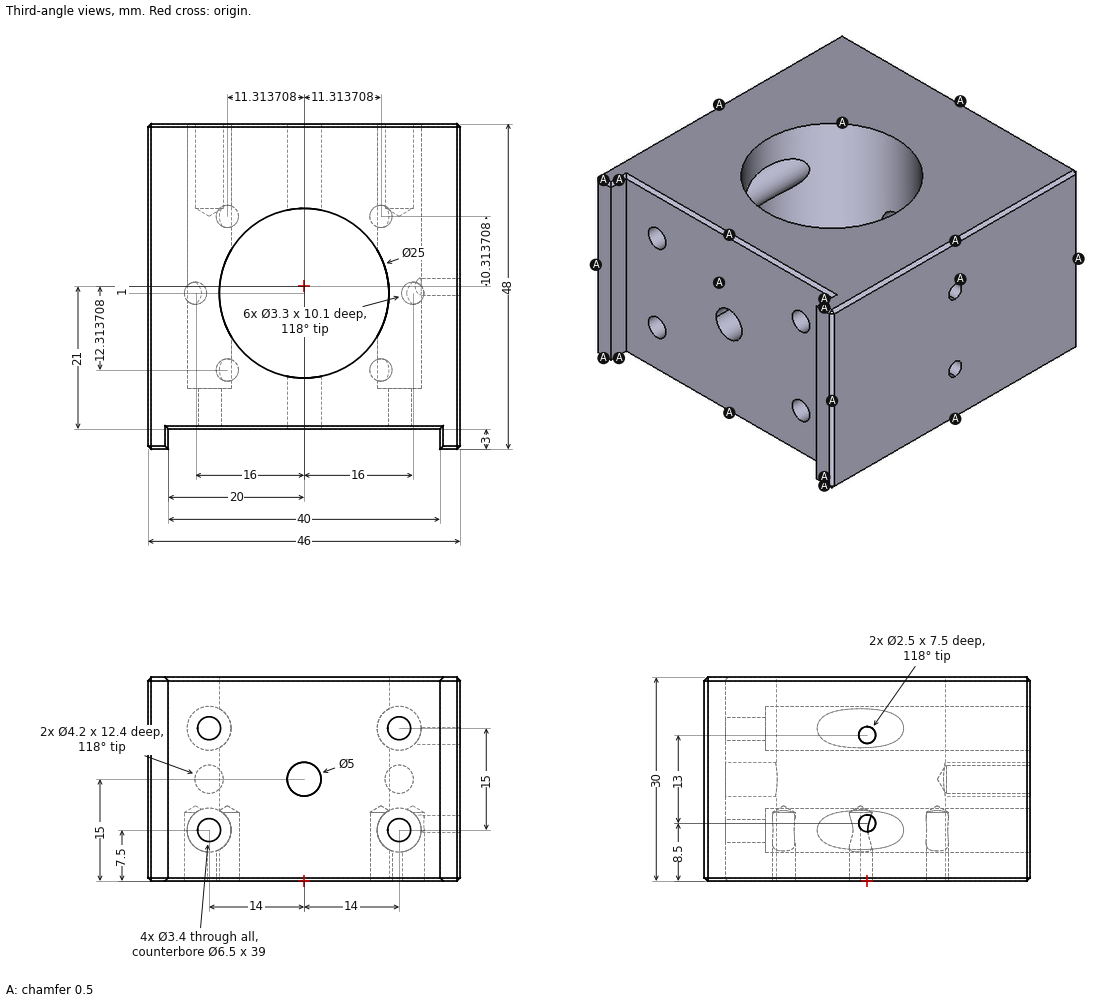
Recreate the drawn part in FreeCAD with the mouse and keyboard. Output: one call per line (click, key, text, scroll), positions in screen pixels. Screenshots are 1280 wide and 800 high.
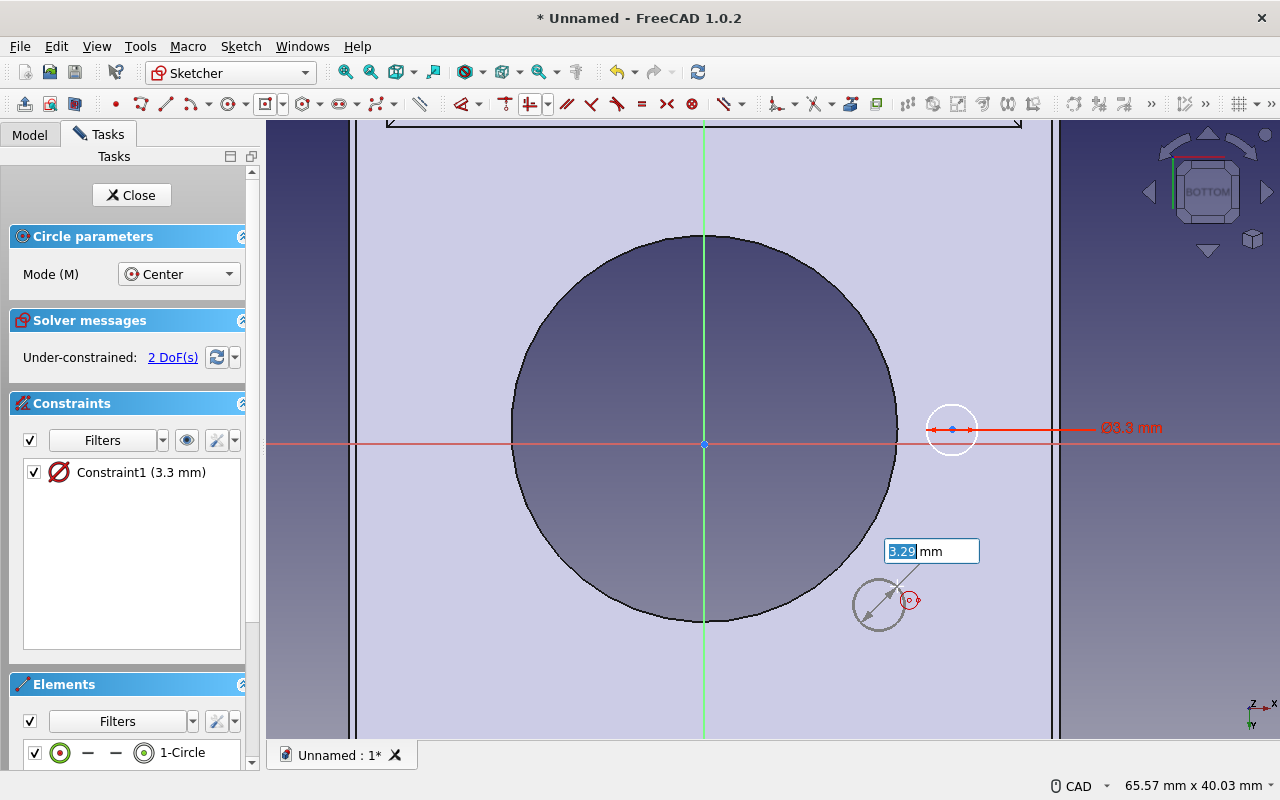
text(3.3)
key(Return)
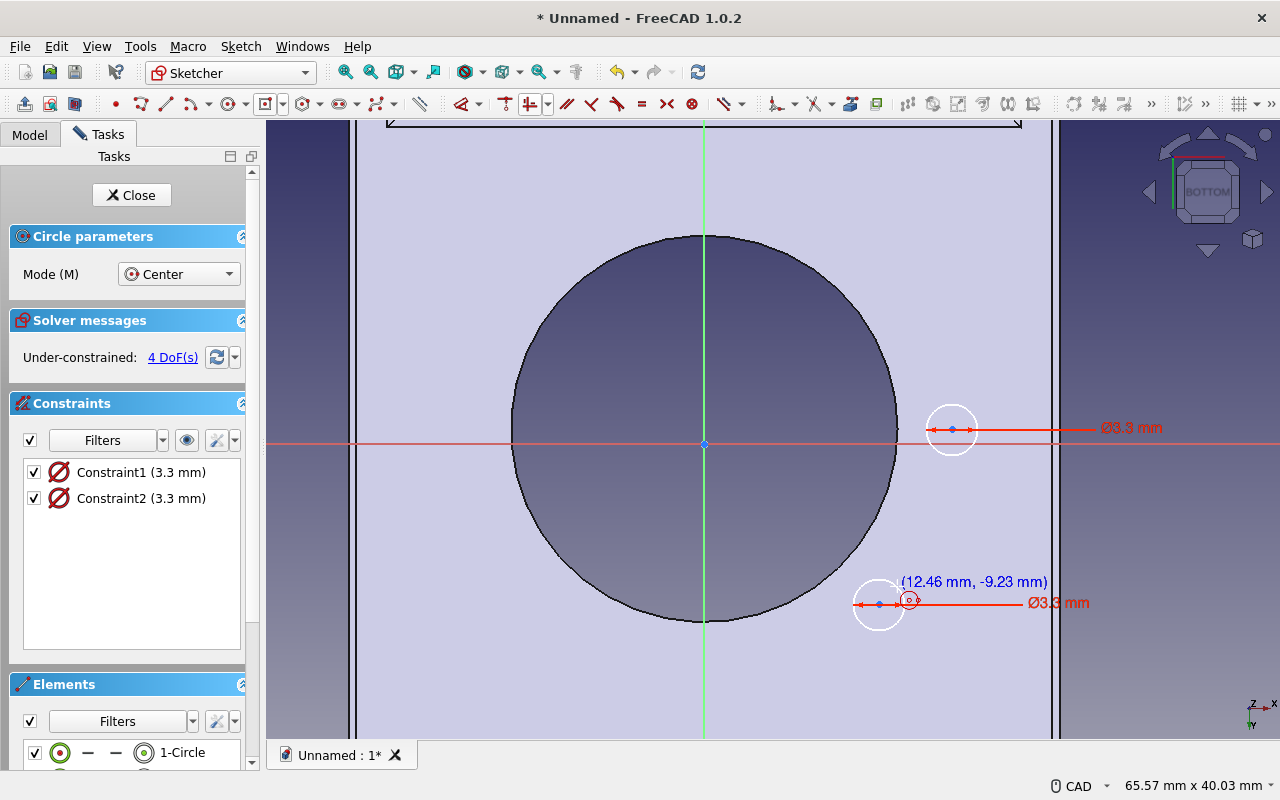
click(529, 604)
move(547, 586)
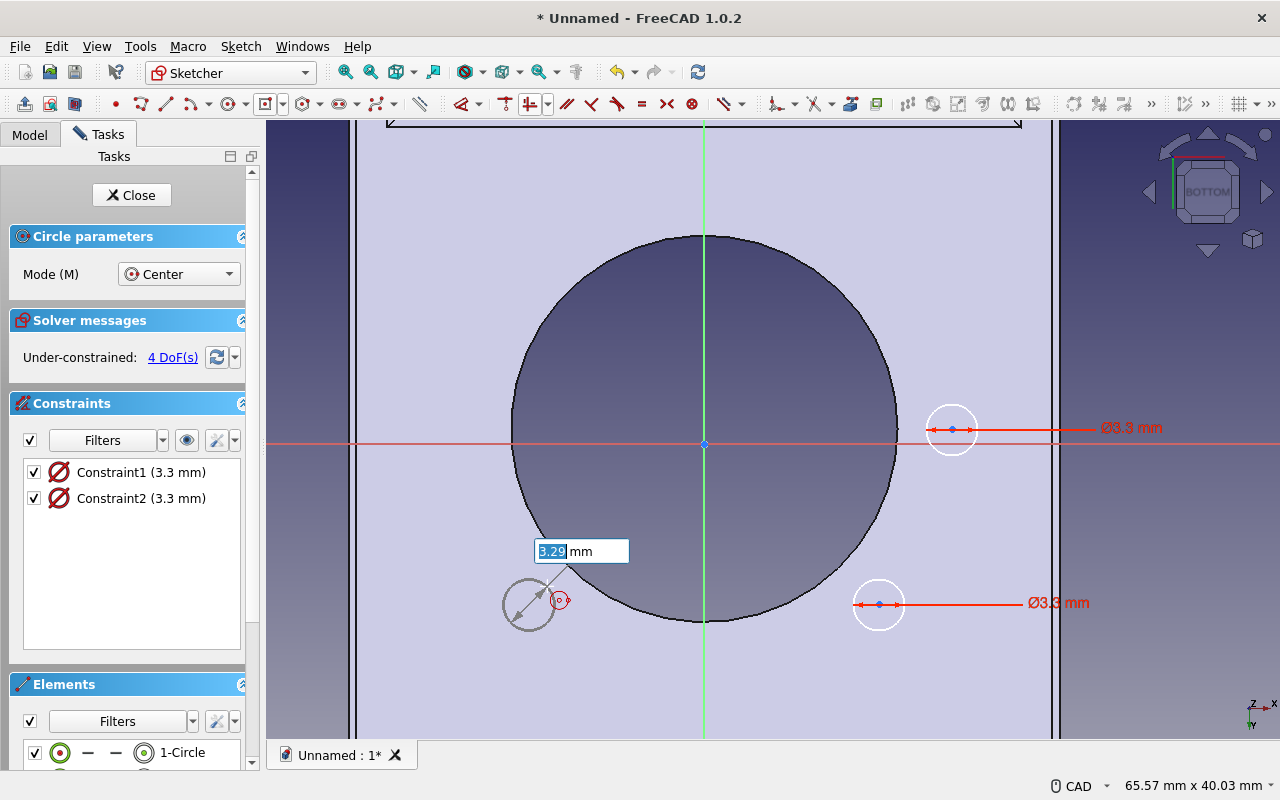
text(3.3)
key(Return)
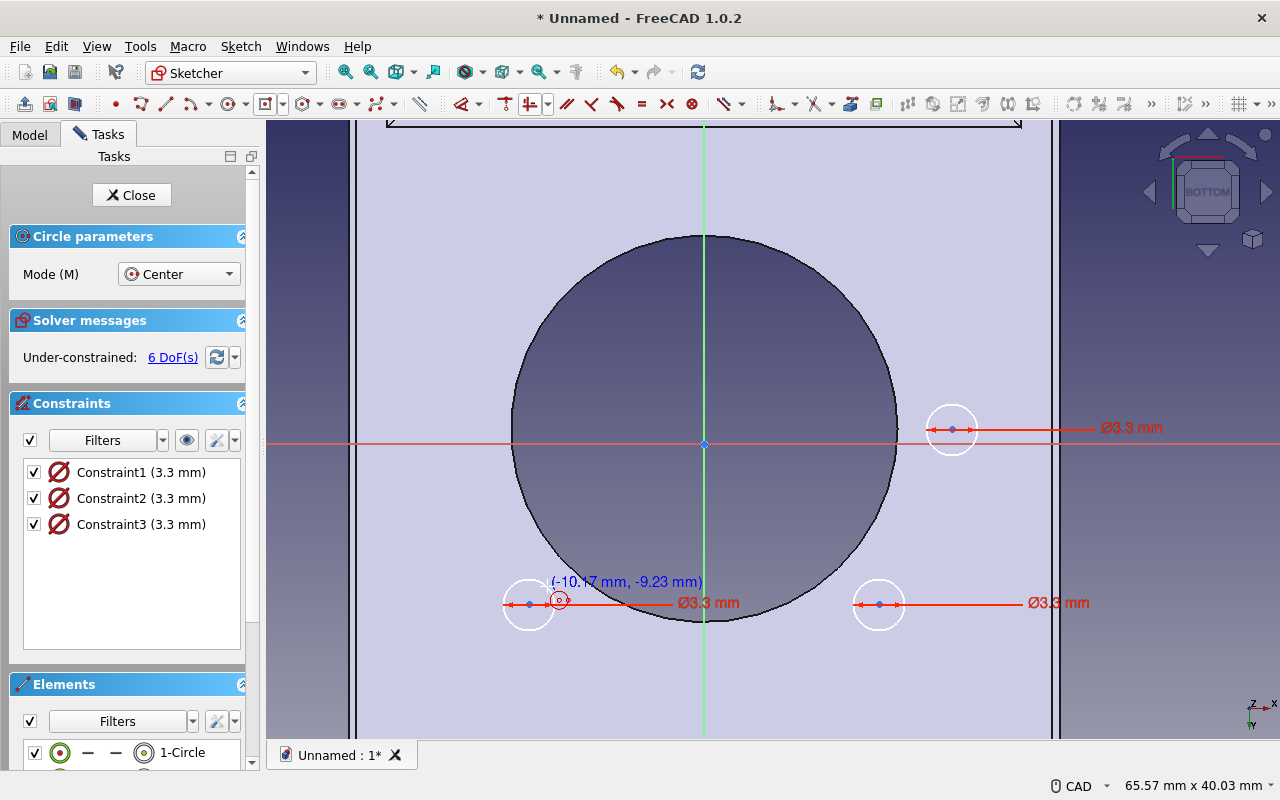
click(457, 429)
move(475, 411)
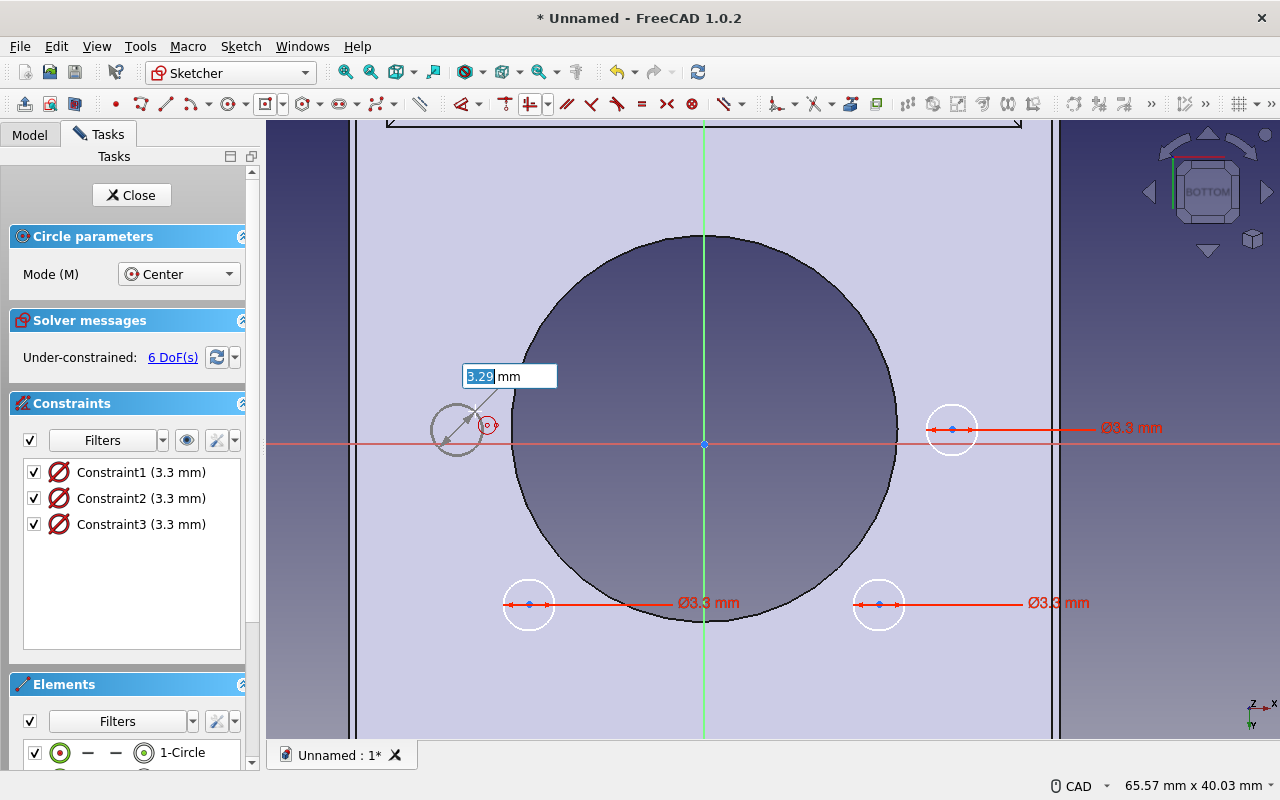
text(3.3)
key(Return)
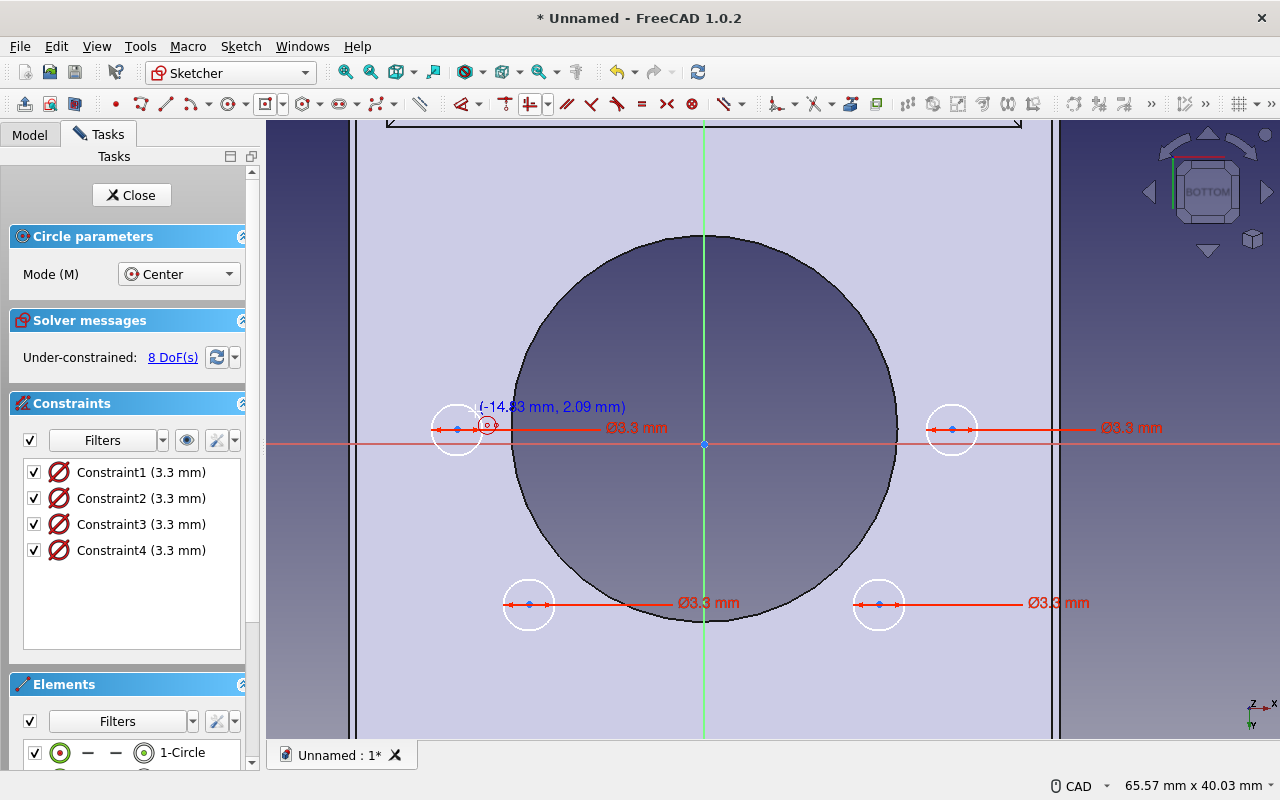
click(529, 254)
move(547, 236)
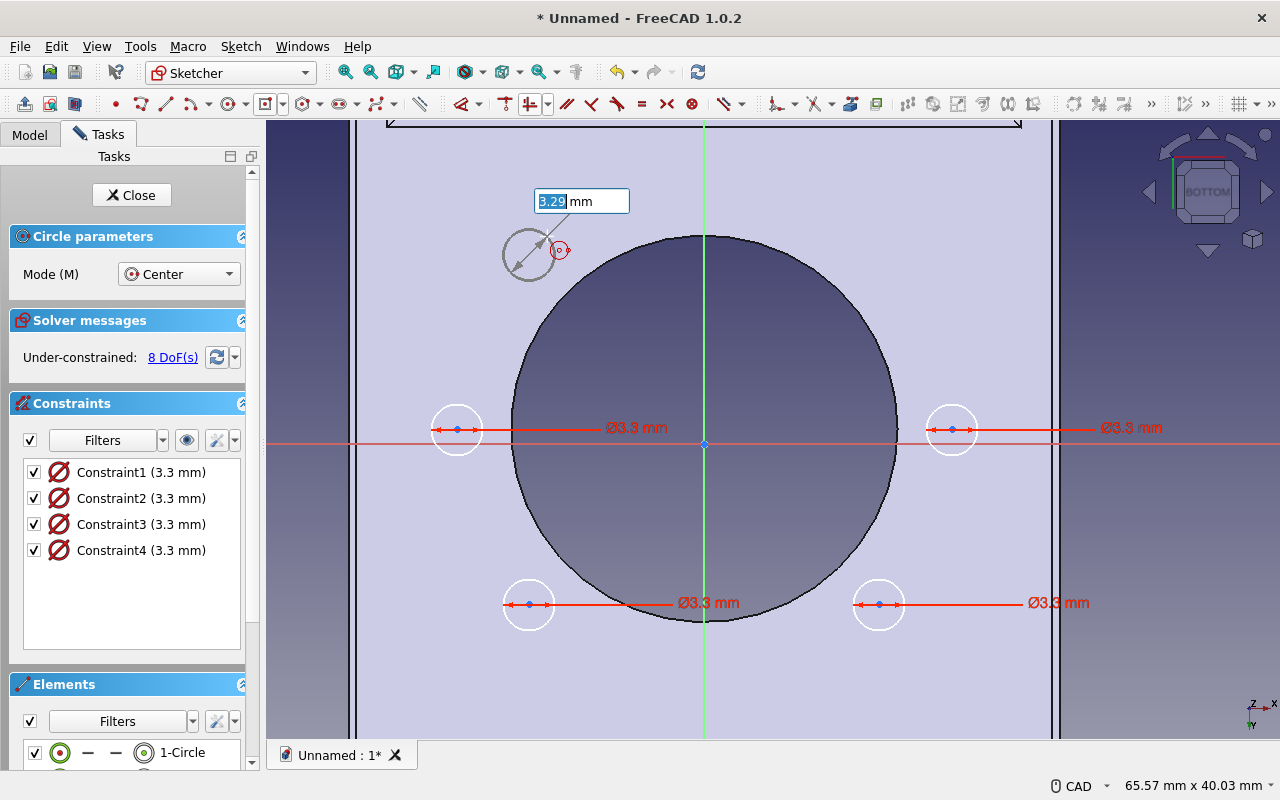
text(3.3)
key(Return)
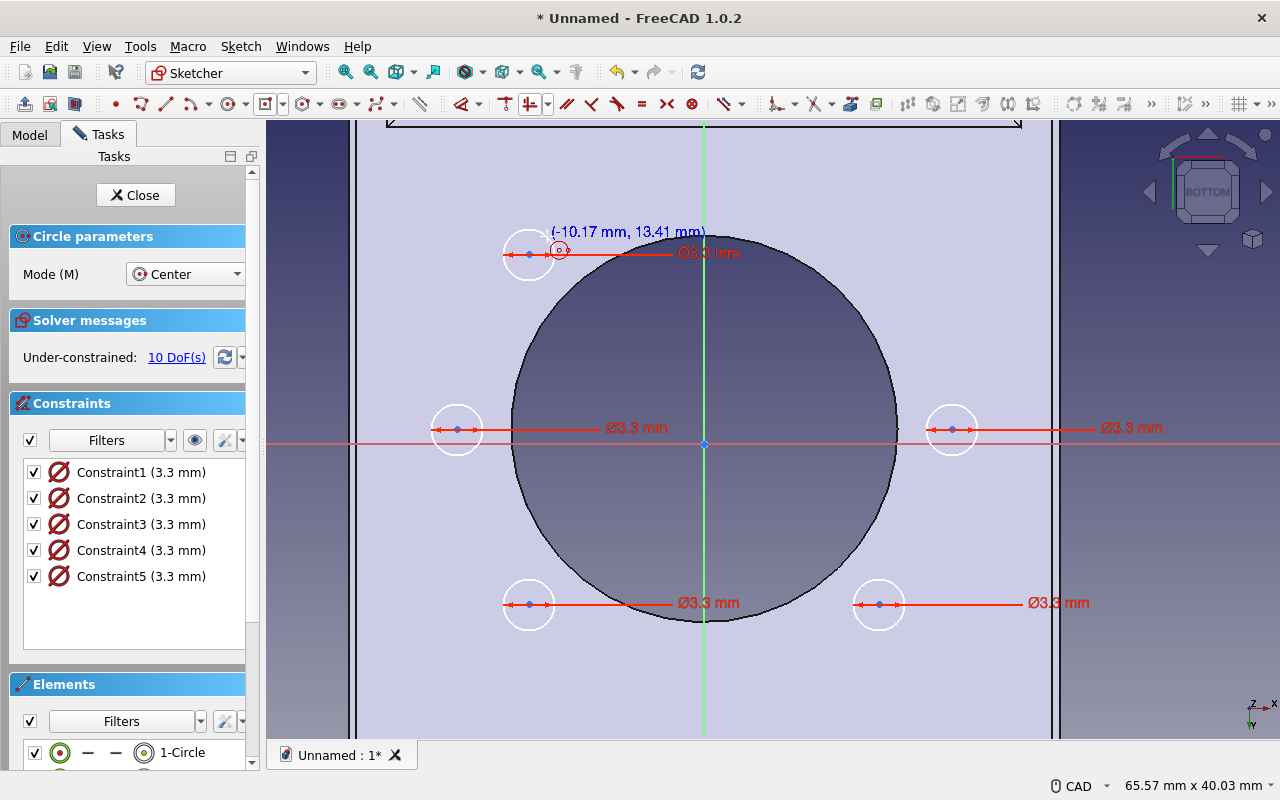
click(879, 254)
move(897, 236)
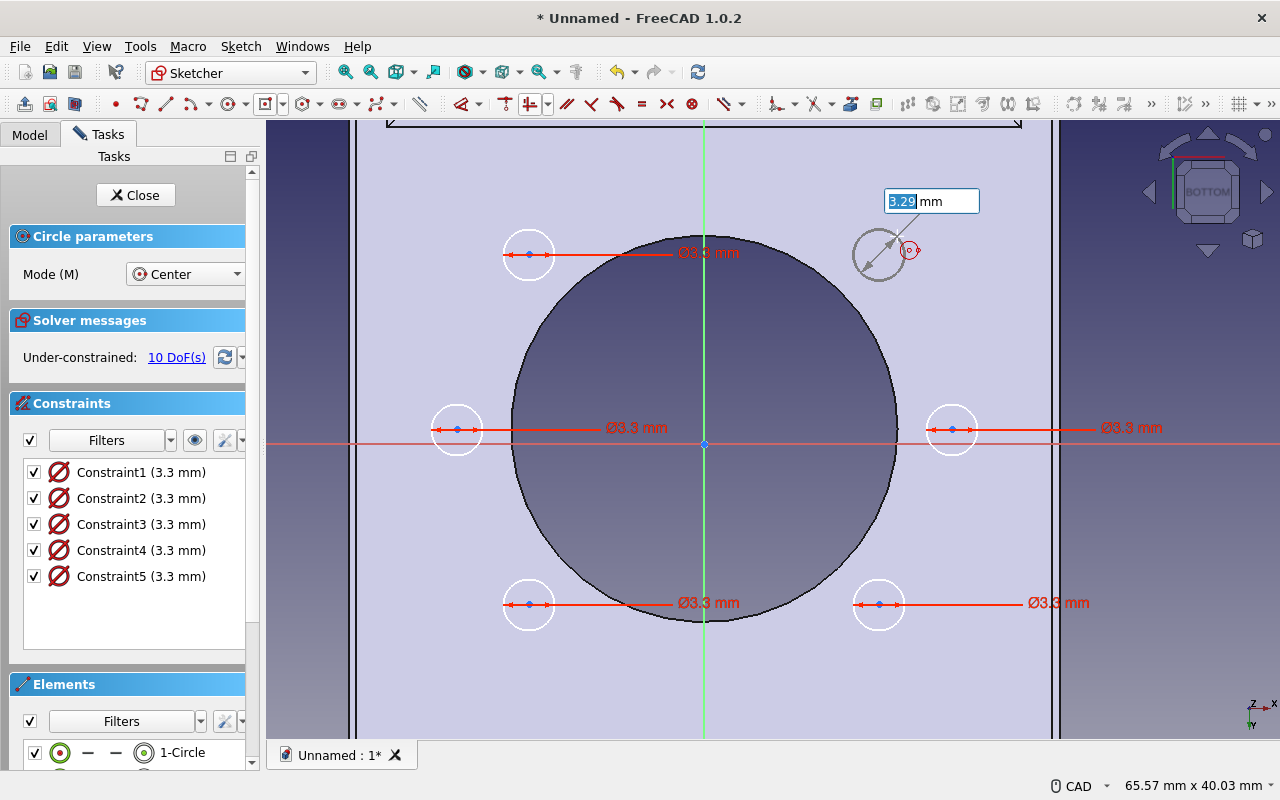
text(3.3)
key(Return)
key(Escape)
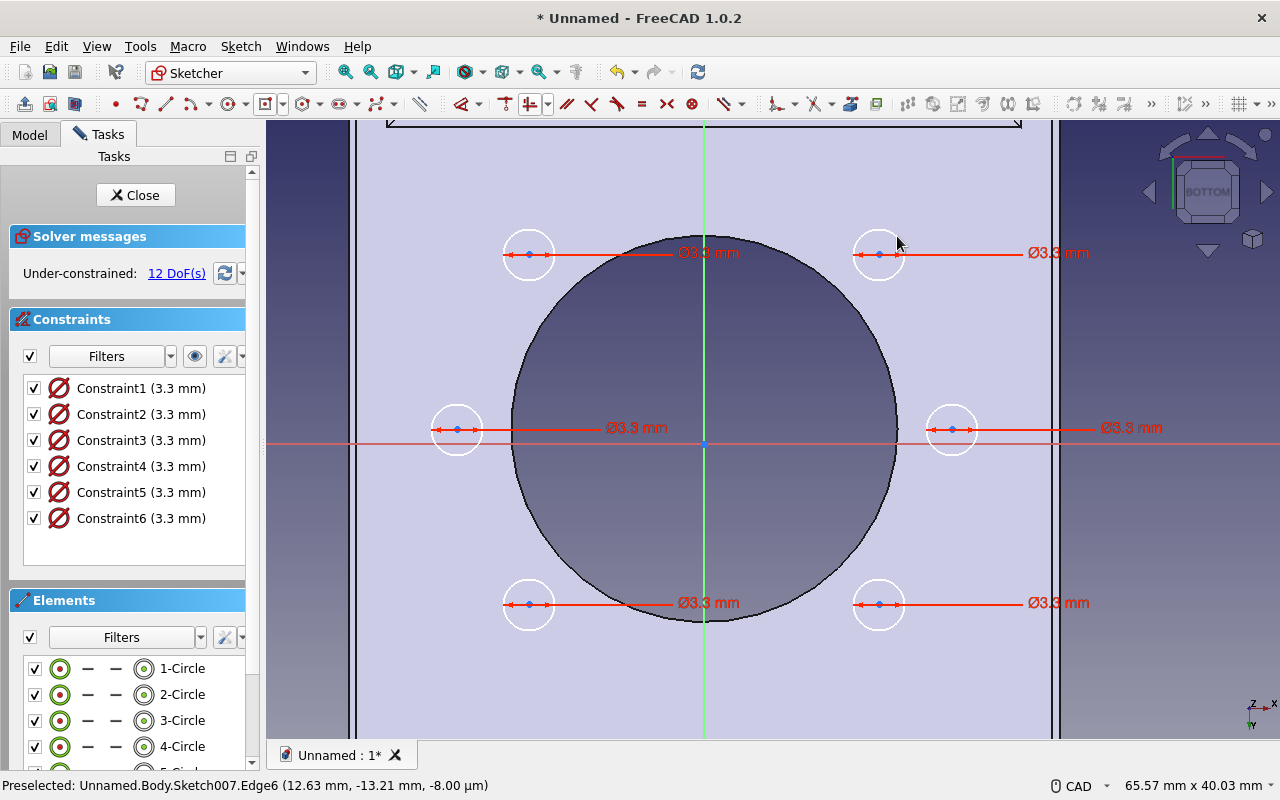
click(879, 605)